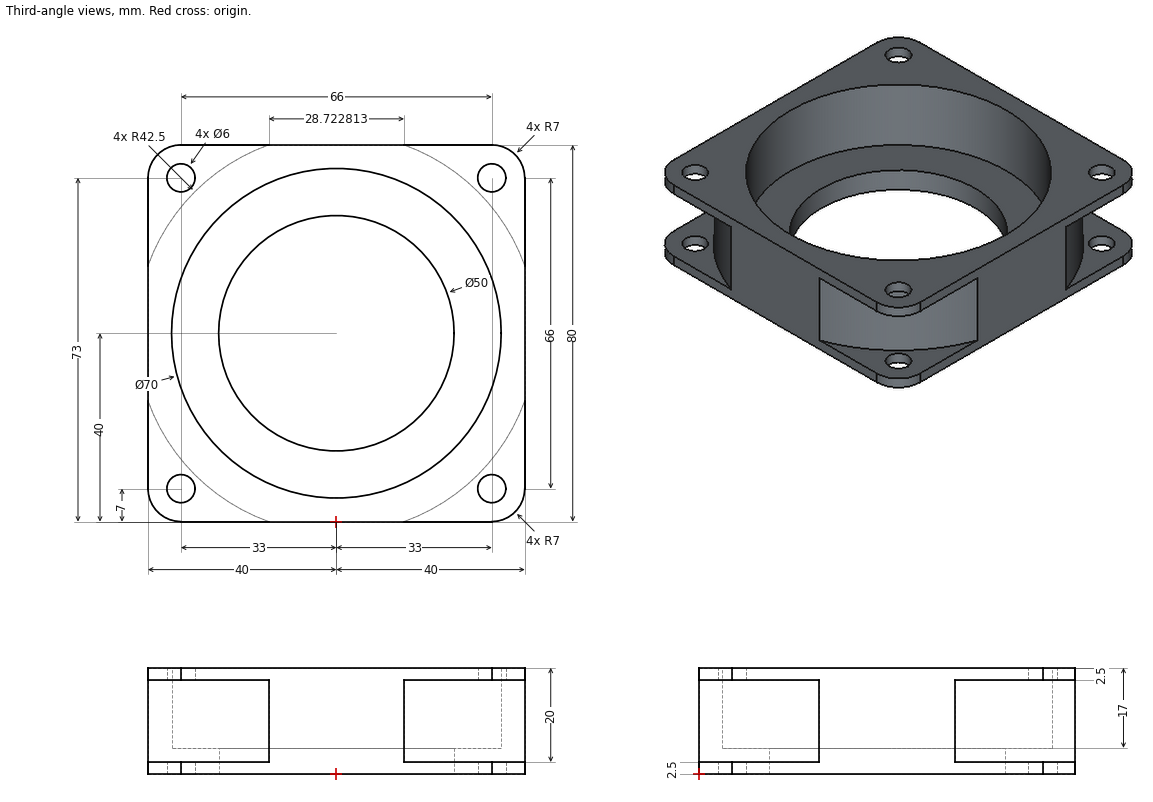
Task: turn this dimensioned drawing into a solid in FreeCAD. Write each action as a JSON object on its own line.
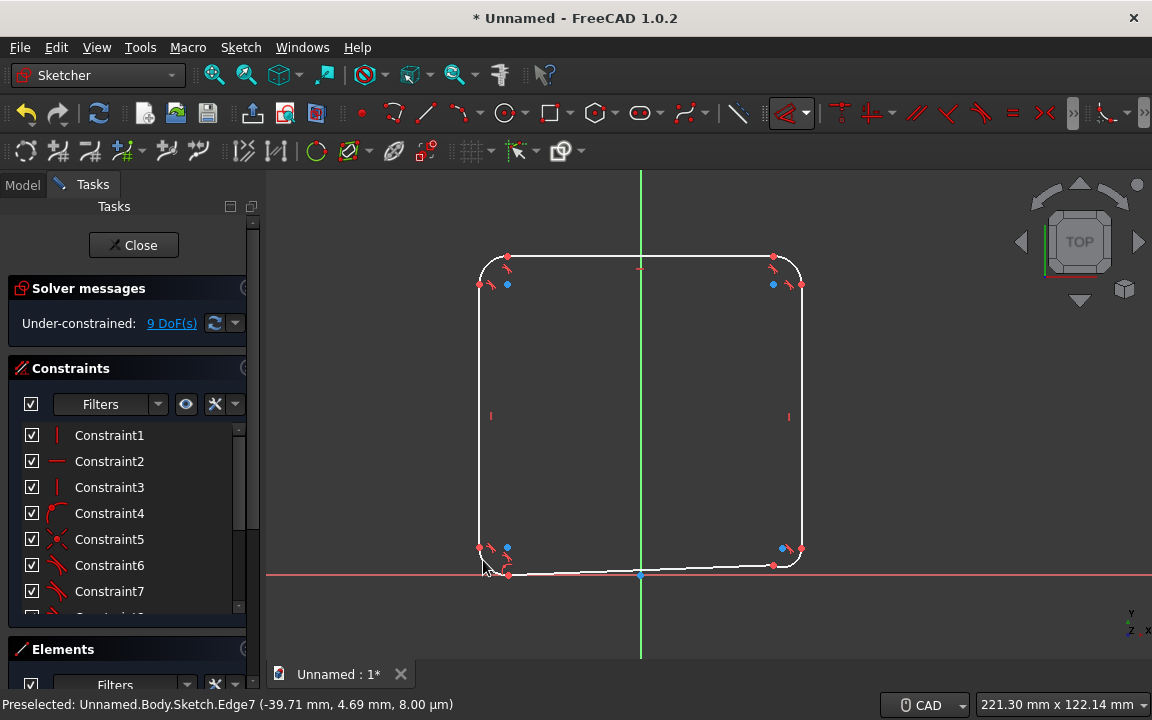
{"action": "left_click", "coordinate": [588, 572]}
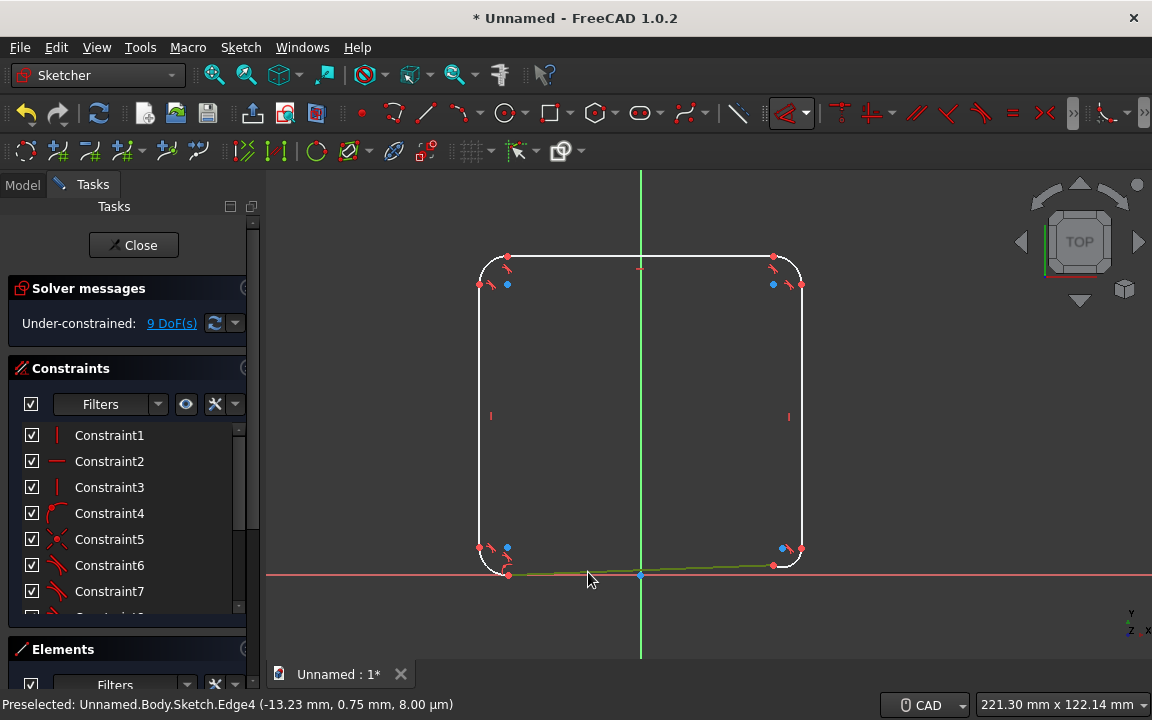
{"action": "left_click", "coordinate": [798, 559]}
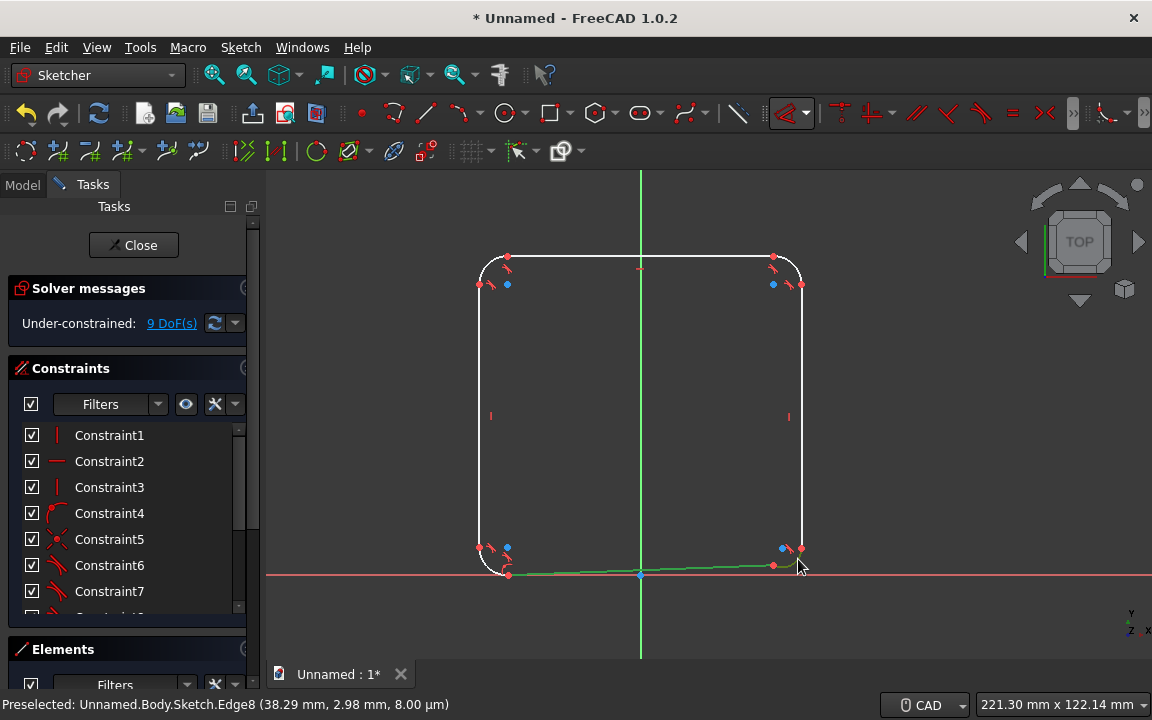
{"action": "key", "text": "t"}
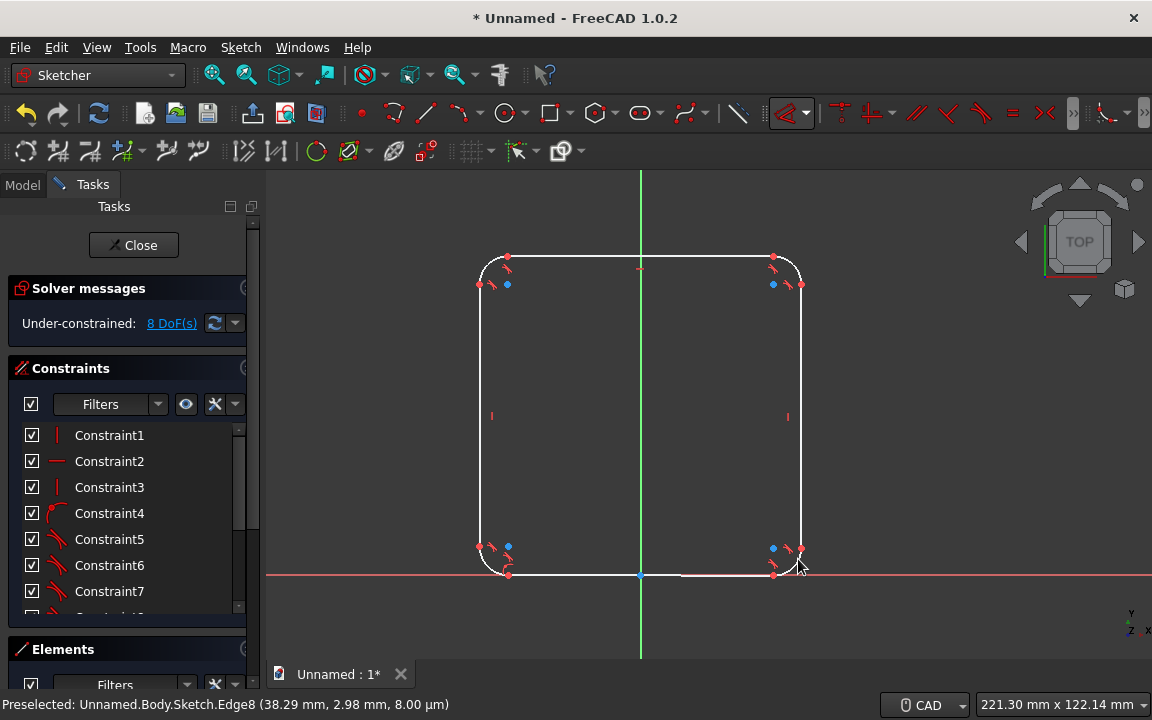
{"action": "left_click", "coordinate": [588, 575]}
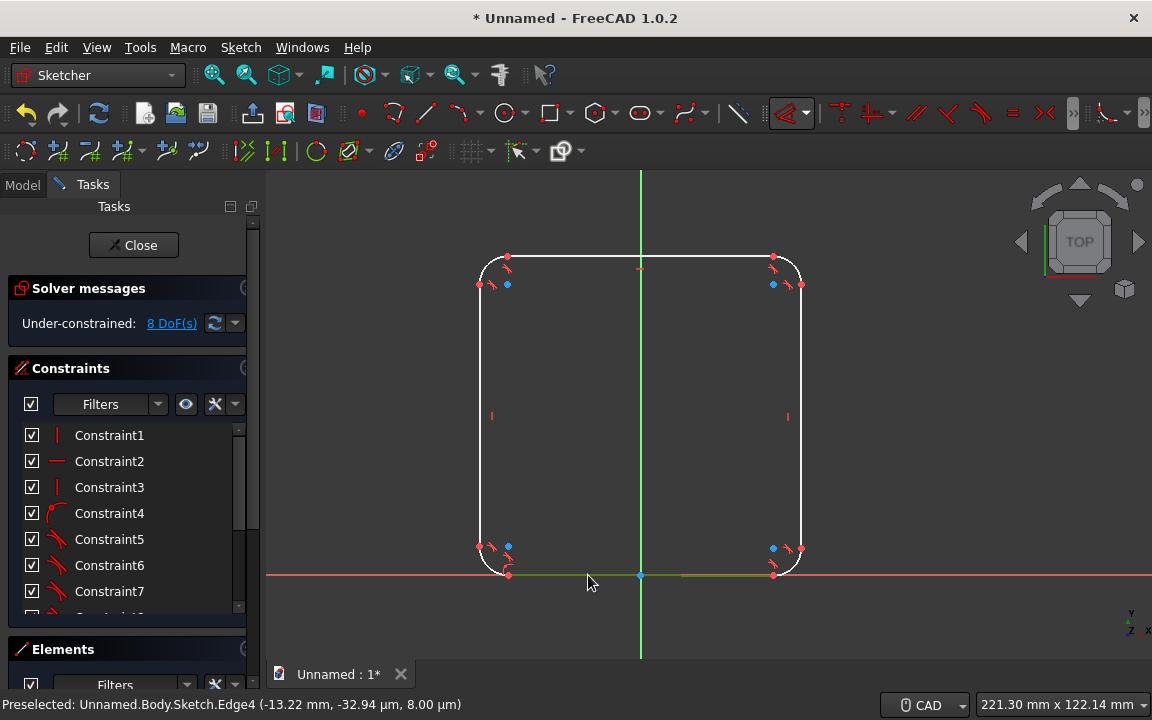
{"action": "key", "text": "h"}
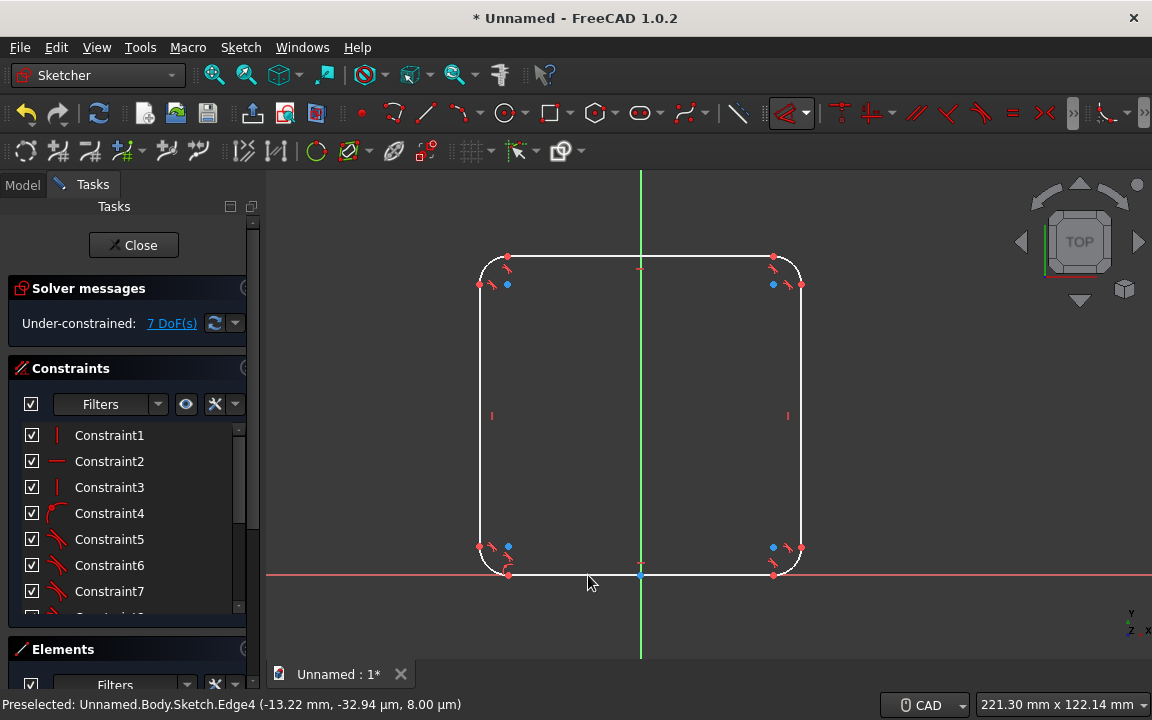
{"action": "left_click", "coordinate": [798, 272]}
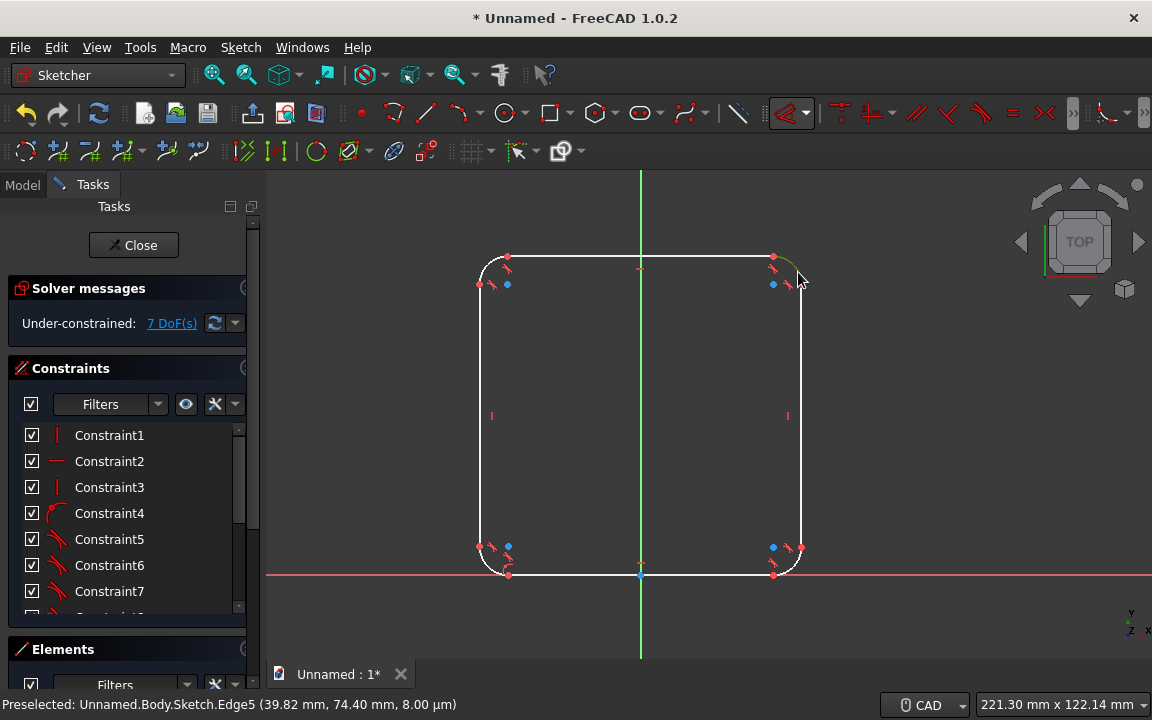
{"action": "left_click", "coordinate": [495, 260]}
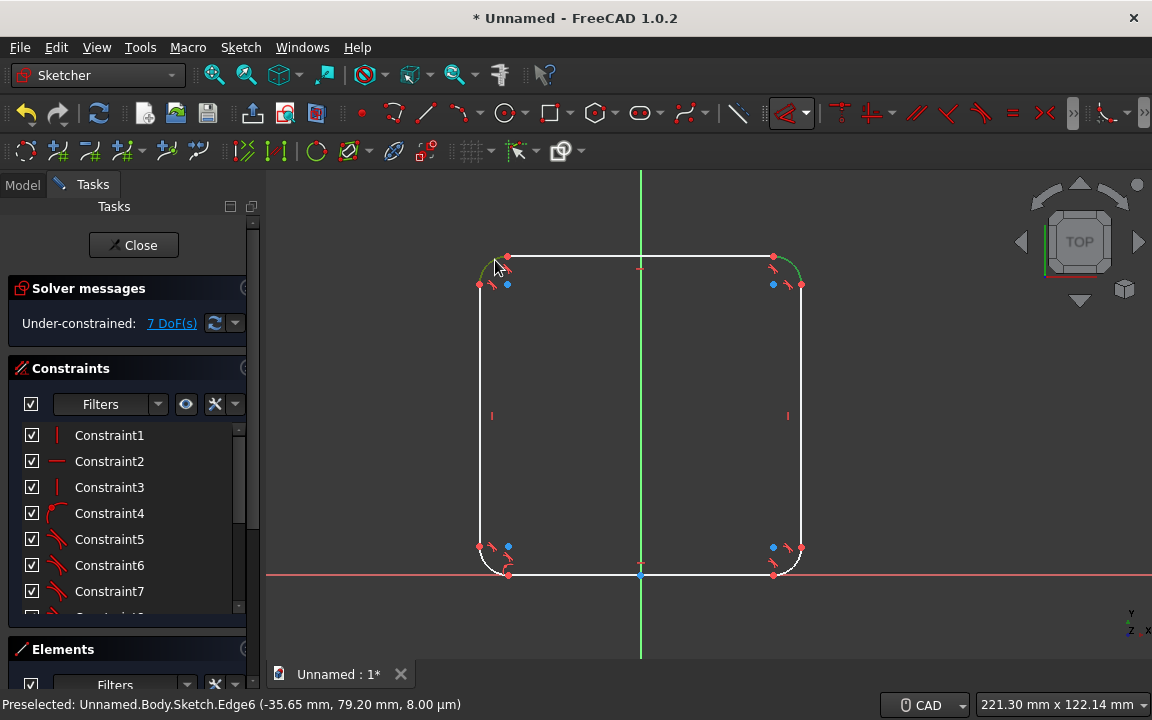
{"action": "left_click", "coordinate": [483, 560]}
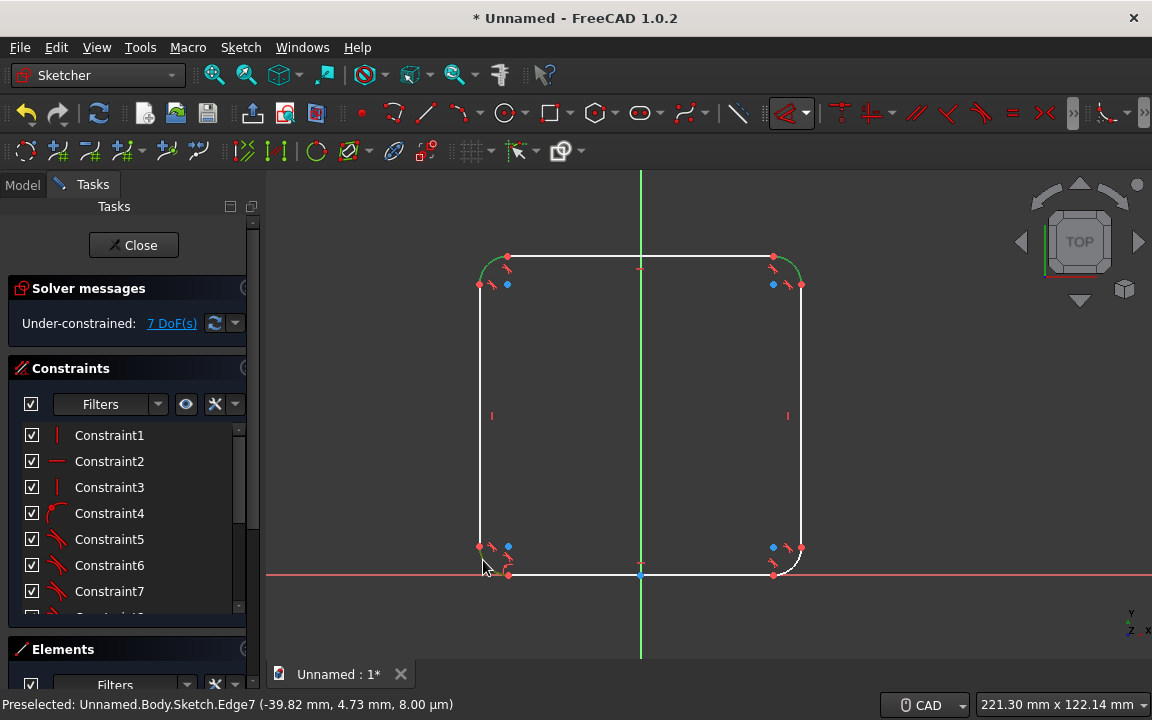
{"action": "left_click", "coordinate": [786, 572]}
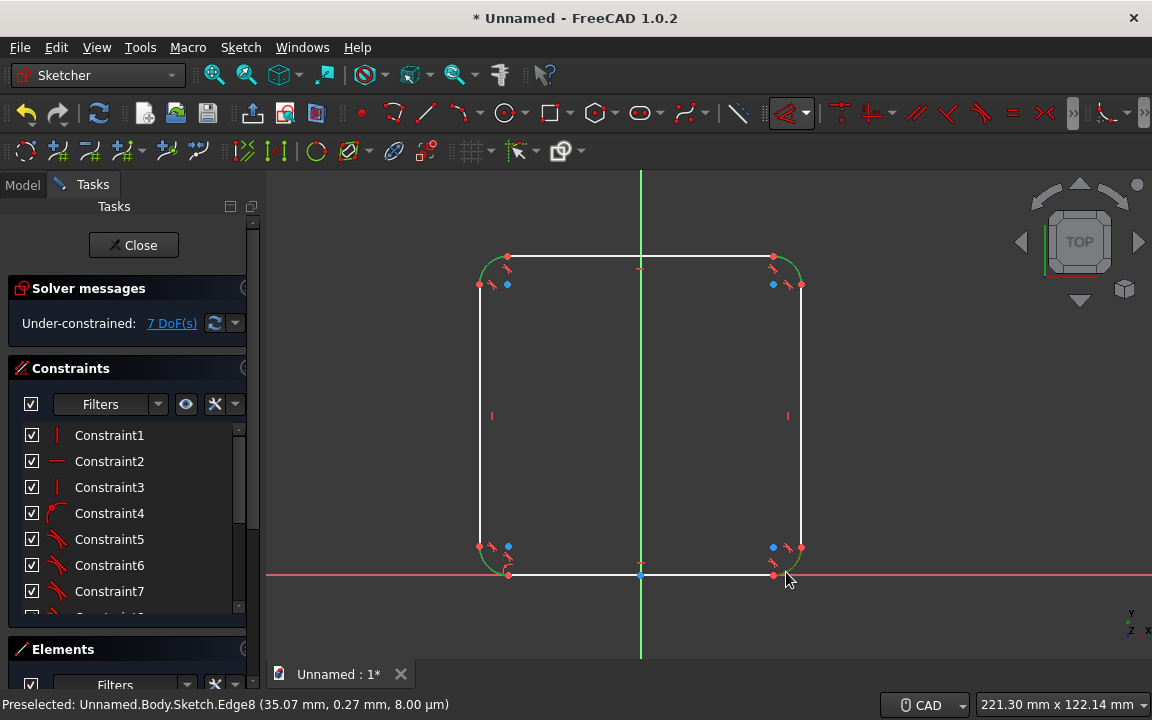
{"action": "key", "text": "e"}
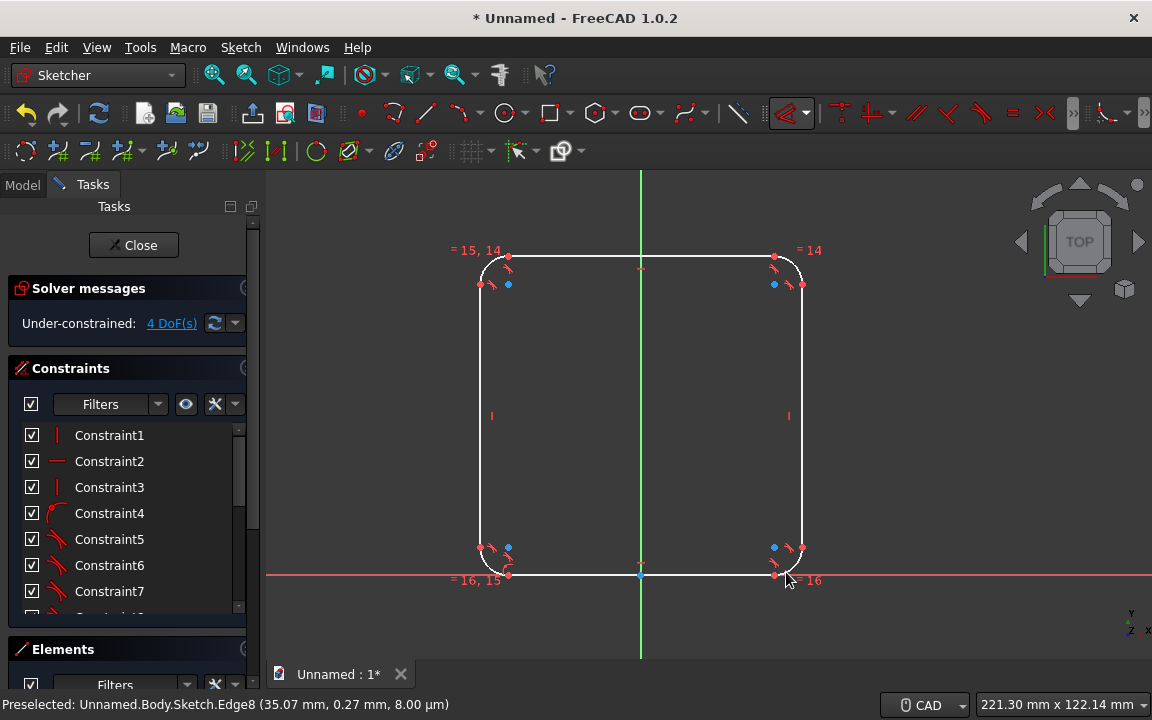
{"action": "key", "text": "d"}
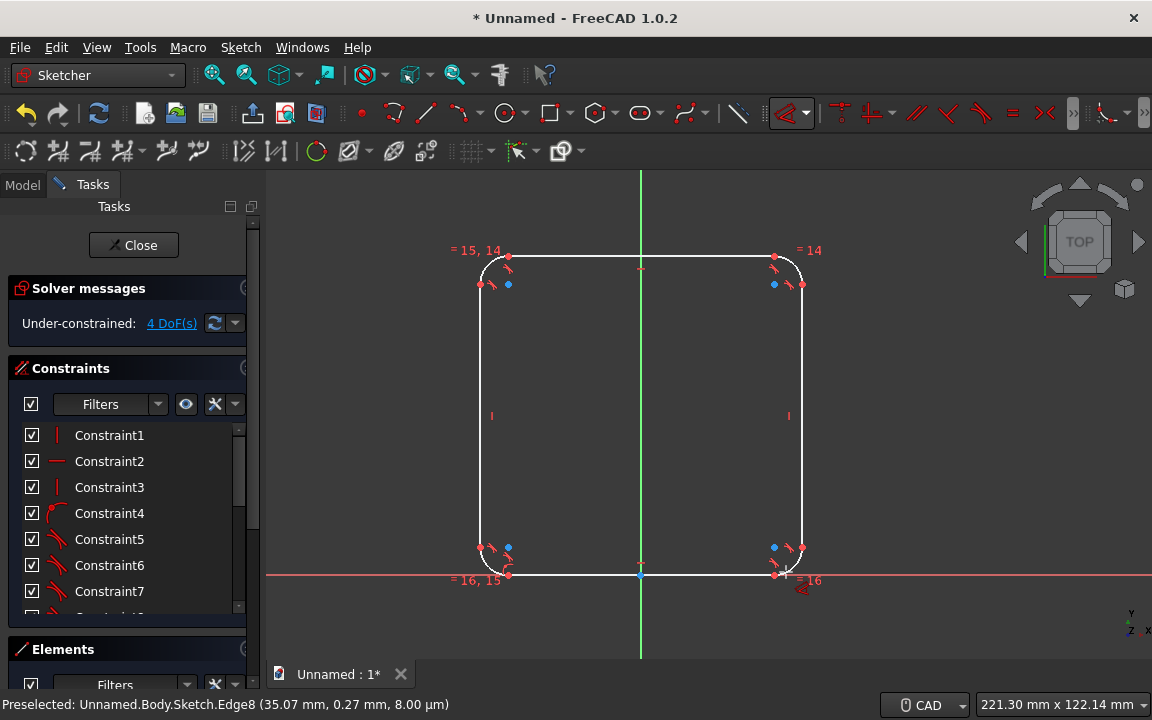
{"action": "scroll", "coordinate": [799, 272], "scroll_direction": "up", "scroll_amount": 2}